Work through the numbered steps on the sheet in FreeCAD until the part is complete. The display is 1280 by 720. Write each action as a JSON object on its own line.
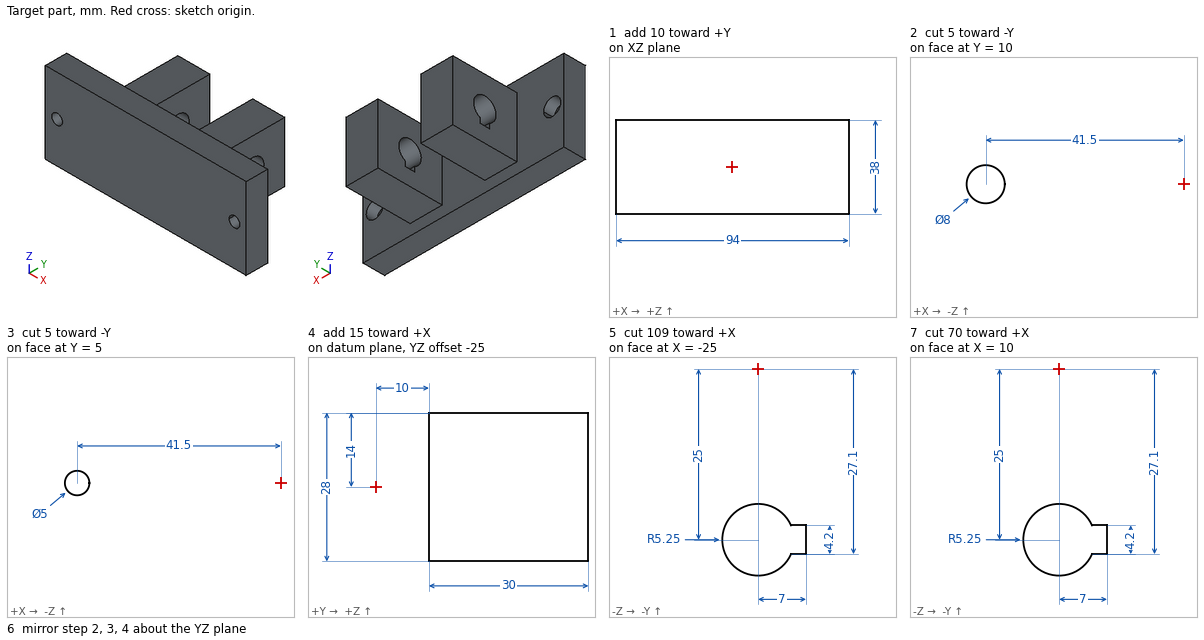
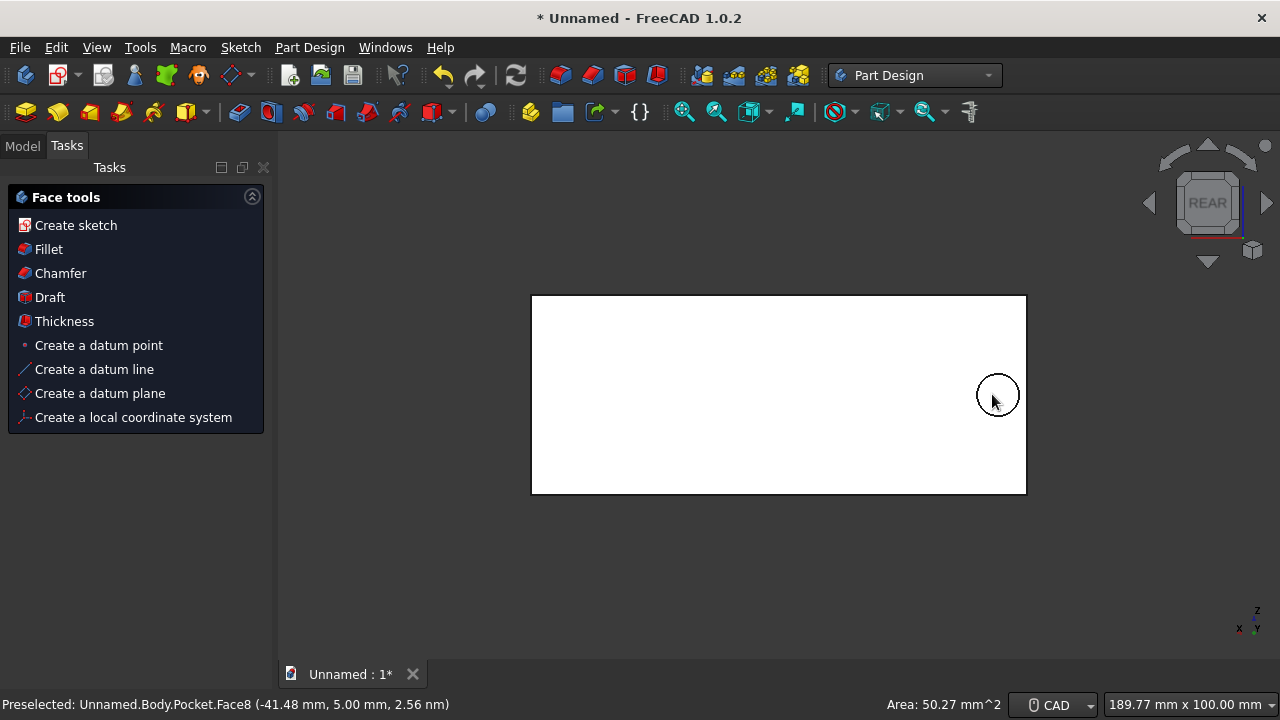
{"action": "left_click", "coordinate": [58, 76]}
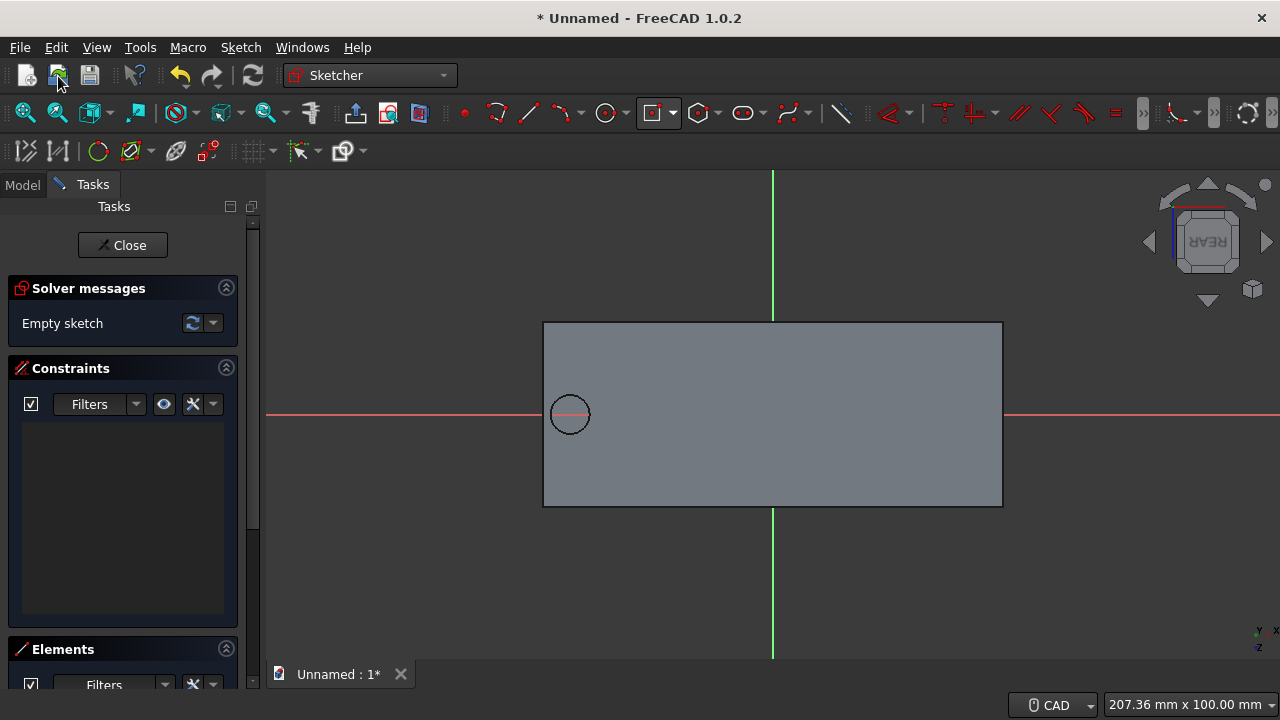
{"action": "left_click", "coordinate": [420, 114]}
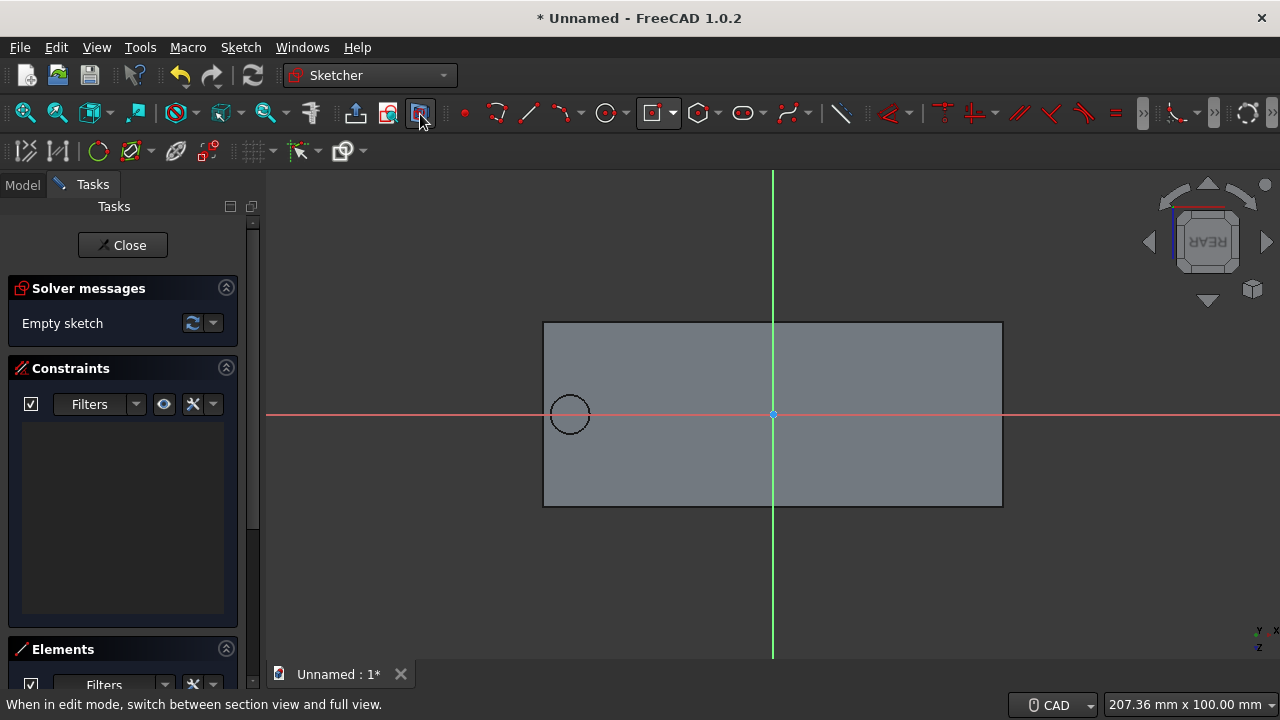
{"action": "scroll", "coordinate": [559, 414], "scroll_direction": "up", "scroll_amount": 13}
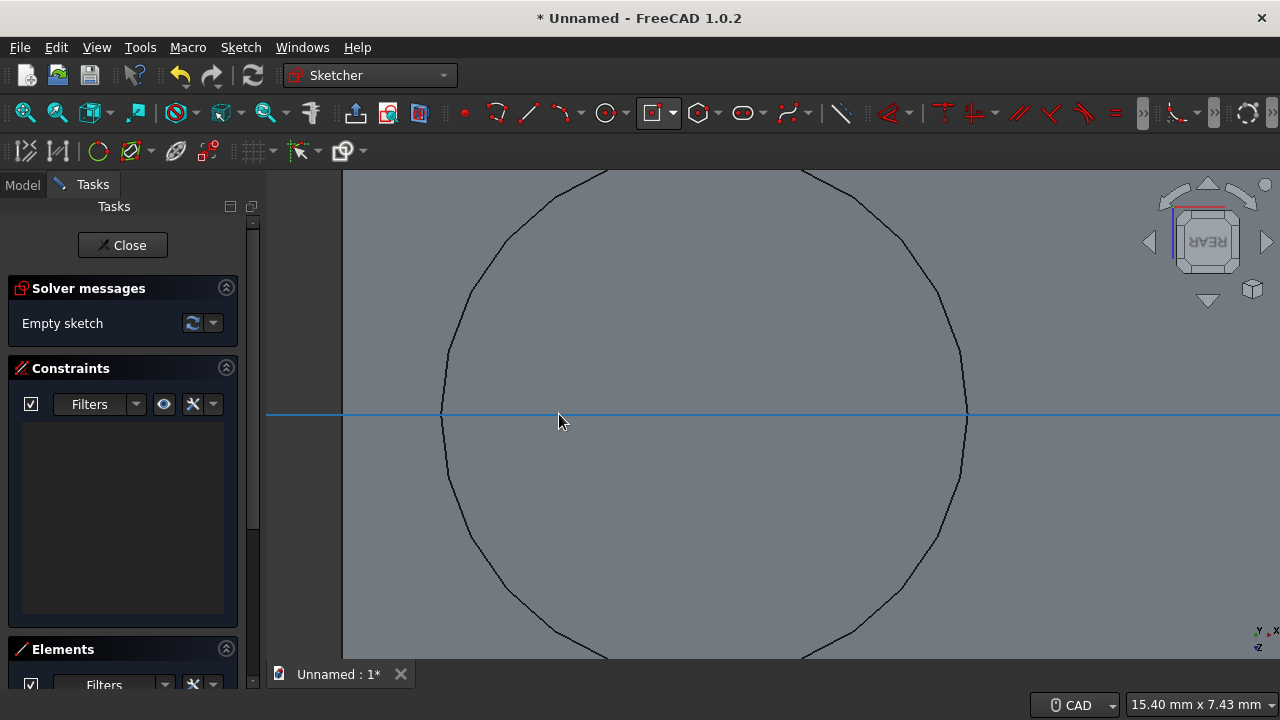
{"action": "left_click", "coordinate": [606, 114]}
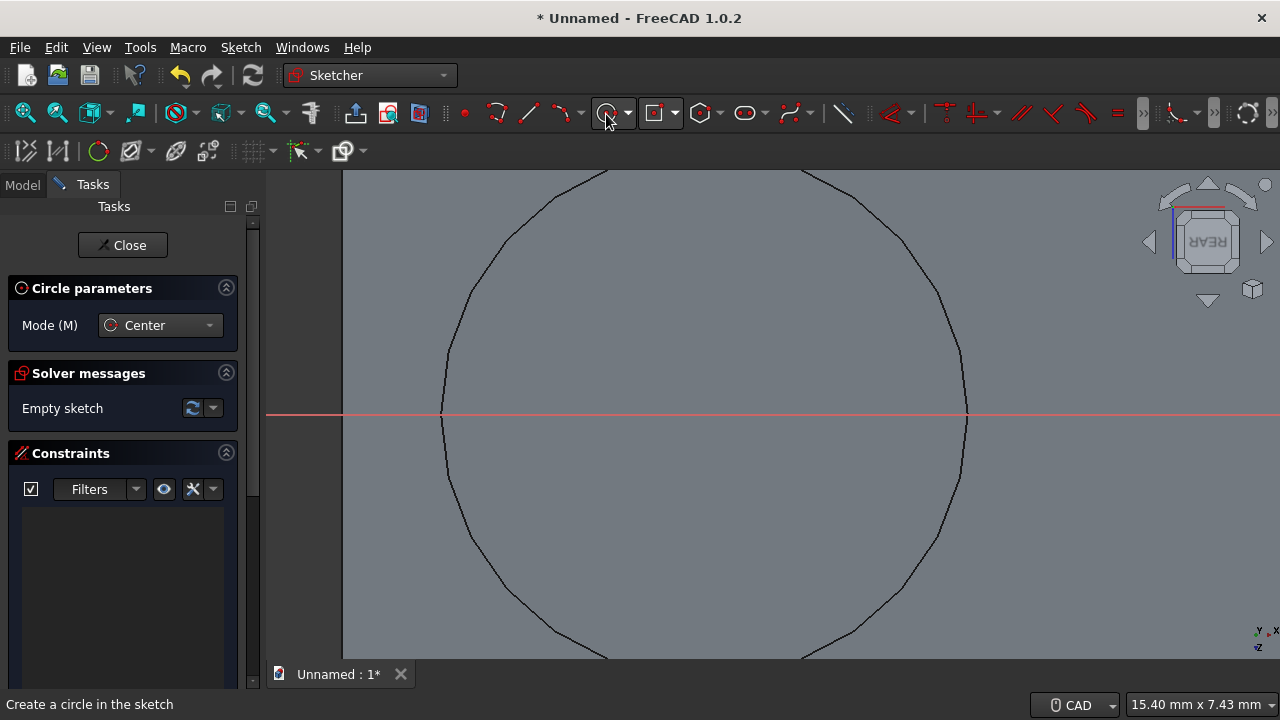
{"action": "left_click", "coordinate": [704, 414]}
{"action": "left_click", "coordinate": [821, 298]}
{"action": "key", "text": "Escape"}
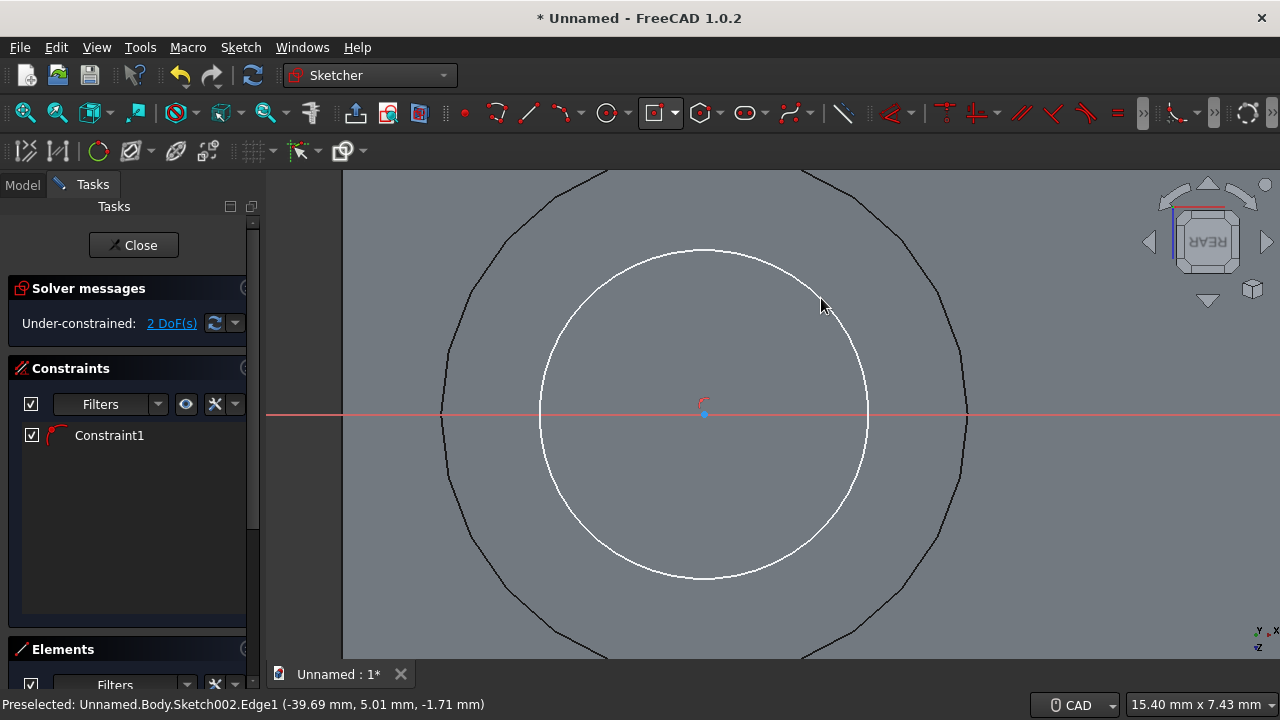
{"action": "left_click", "coordinate": [890, 114]}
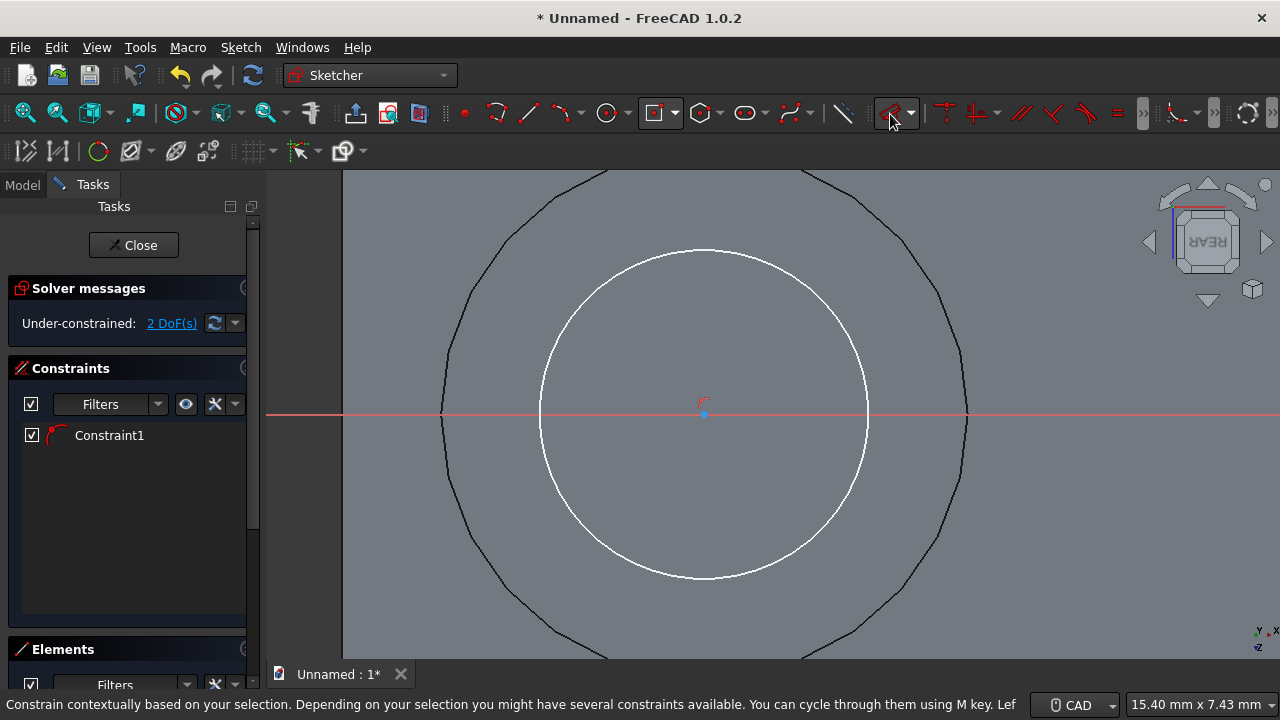
{"action": "left_click", "coordinate": [820, 298]}
{"action": "left_click", "coordinate": [843, 275]}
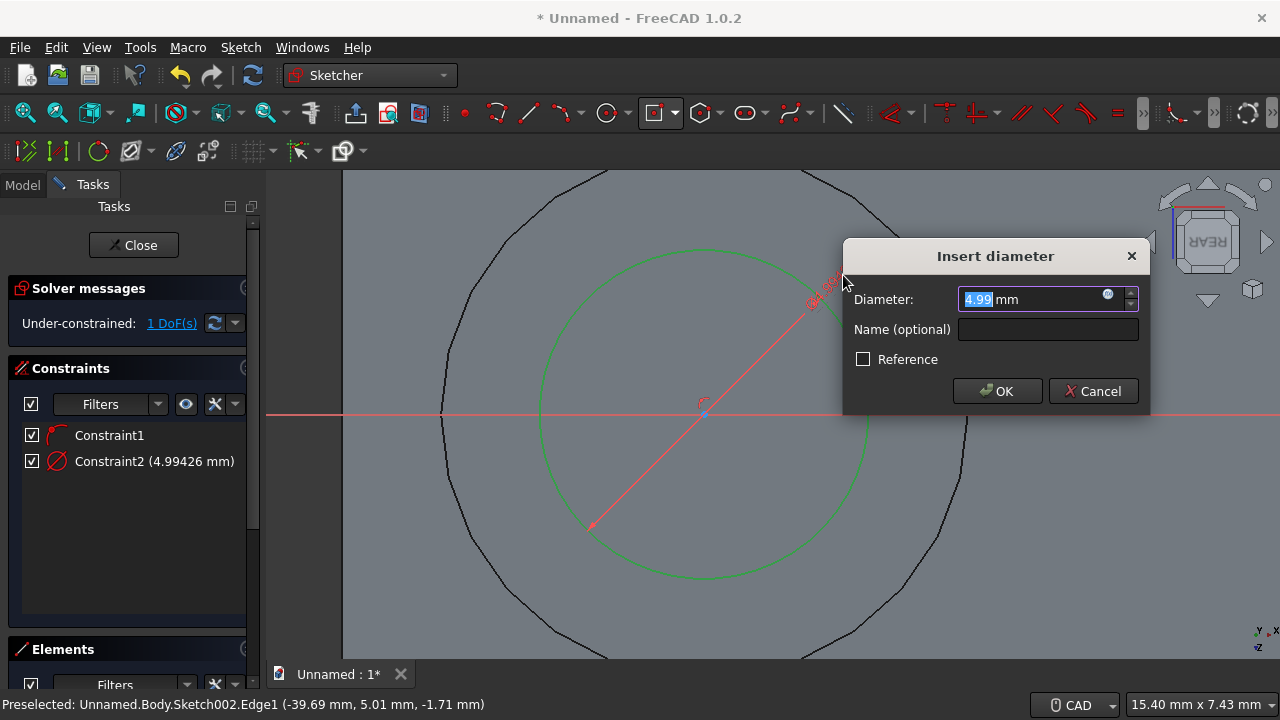
{"action": "type", "text": "5"}
{"action": "key", "text": "Return"}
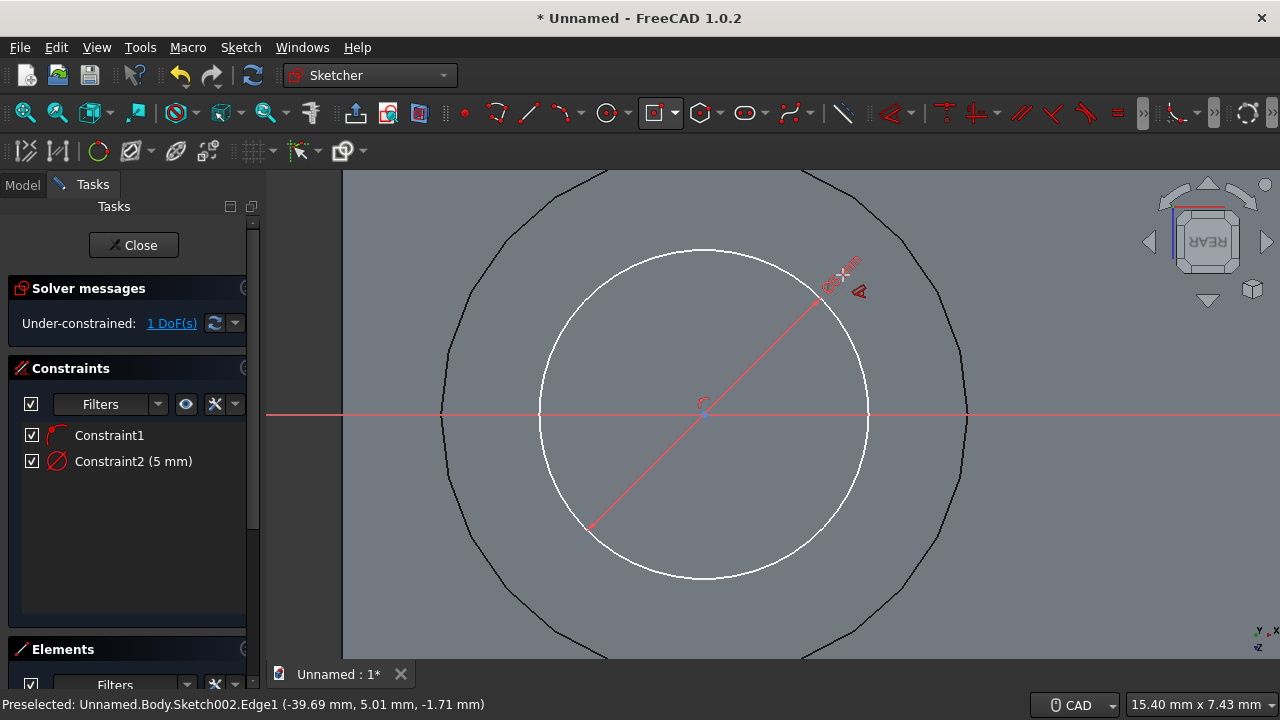
{"action": "left_click", "coordinate": [704, 414]}
{"action": "left_click", "coordinate": [910, 448]}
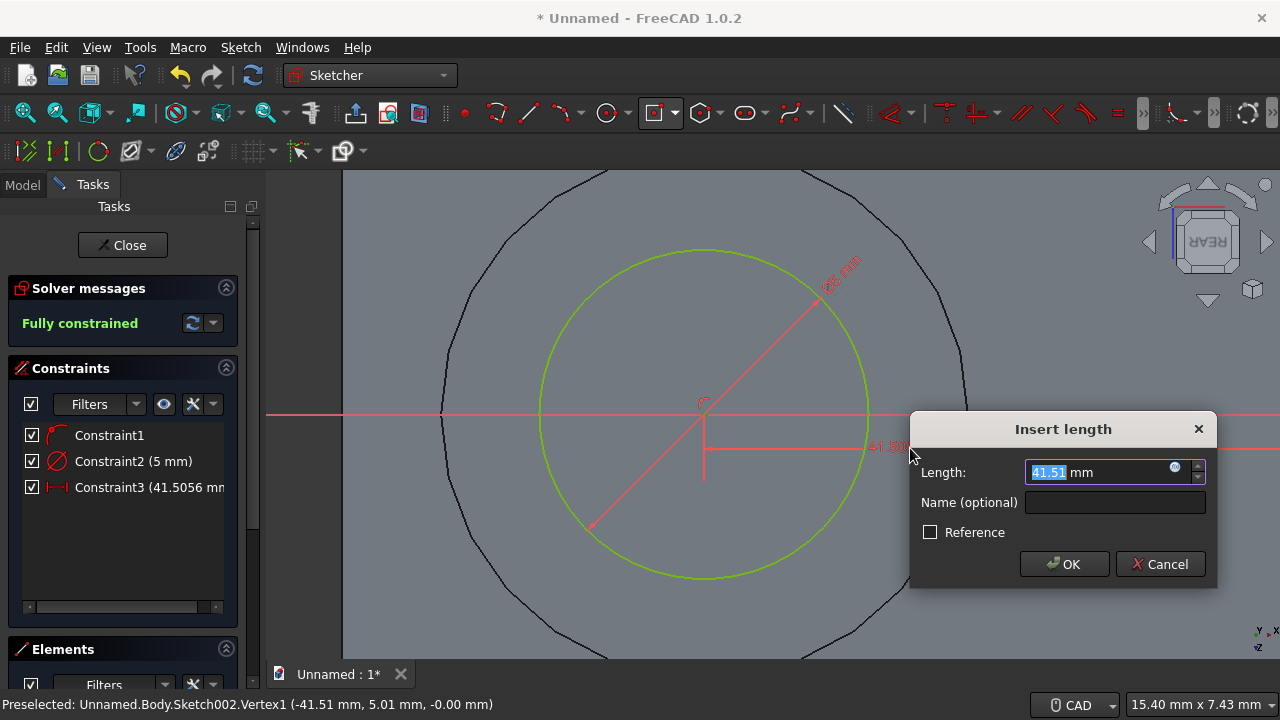
{"action": "type", "text": "41.5"}
{"action": "key", "text": "Return"}
{"action": "key", "text": "Escape"}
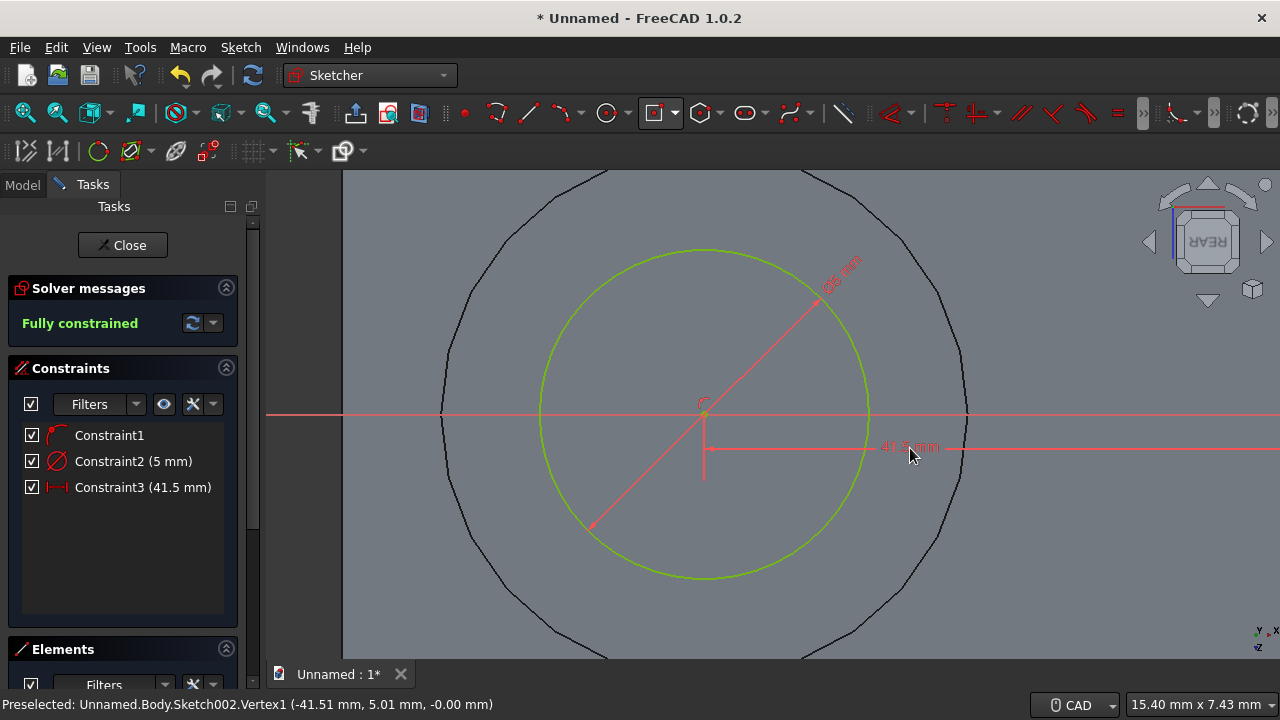
{"action": "left_click", "coordinate": [123, 245]}